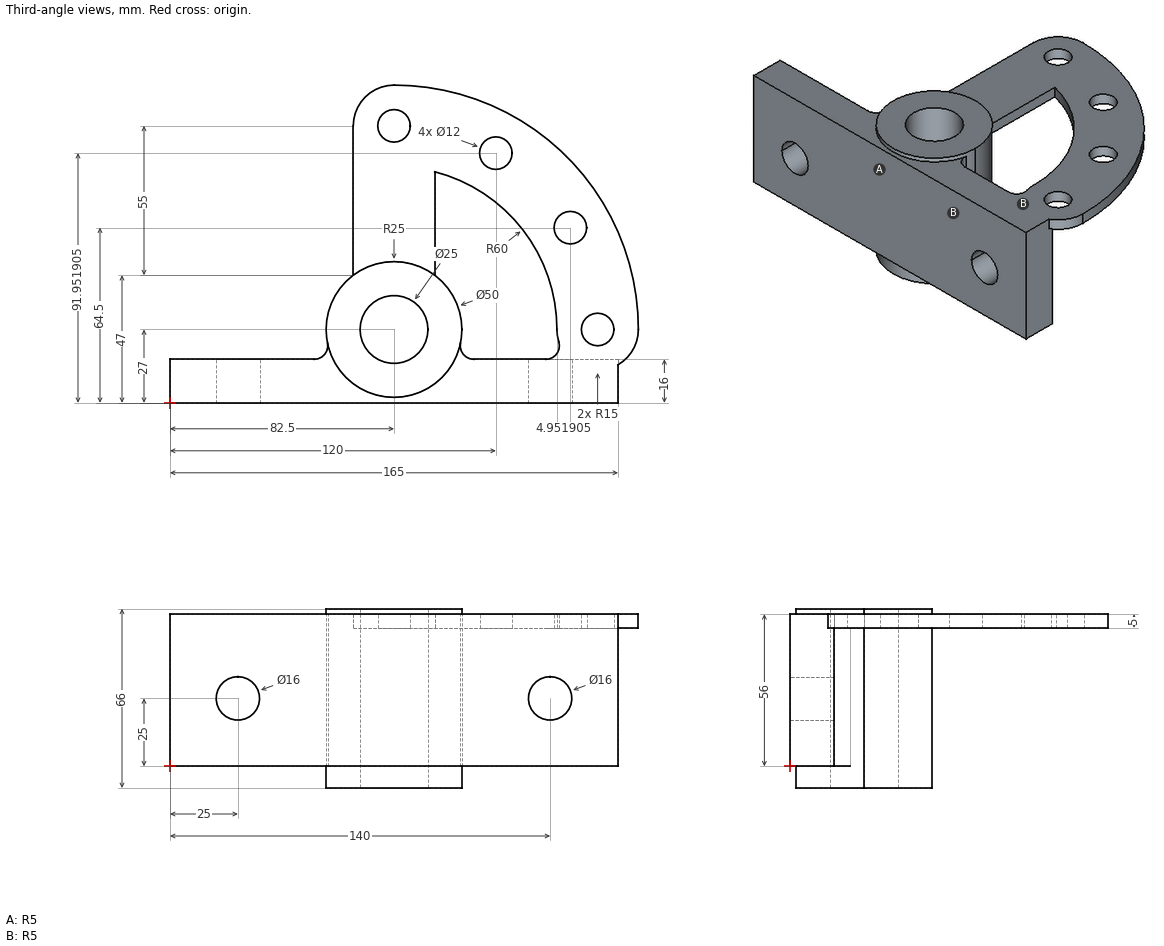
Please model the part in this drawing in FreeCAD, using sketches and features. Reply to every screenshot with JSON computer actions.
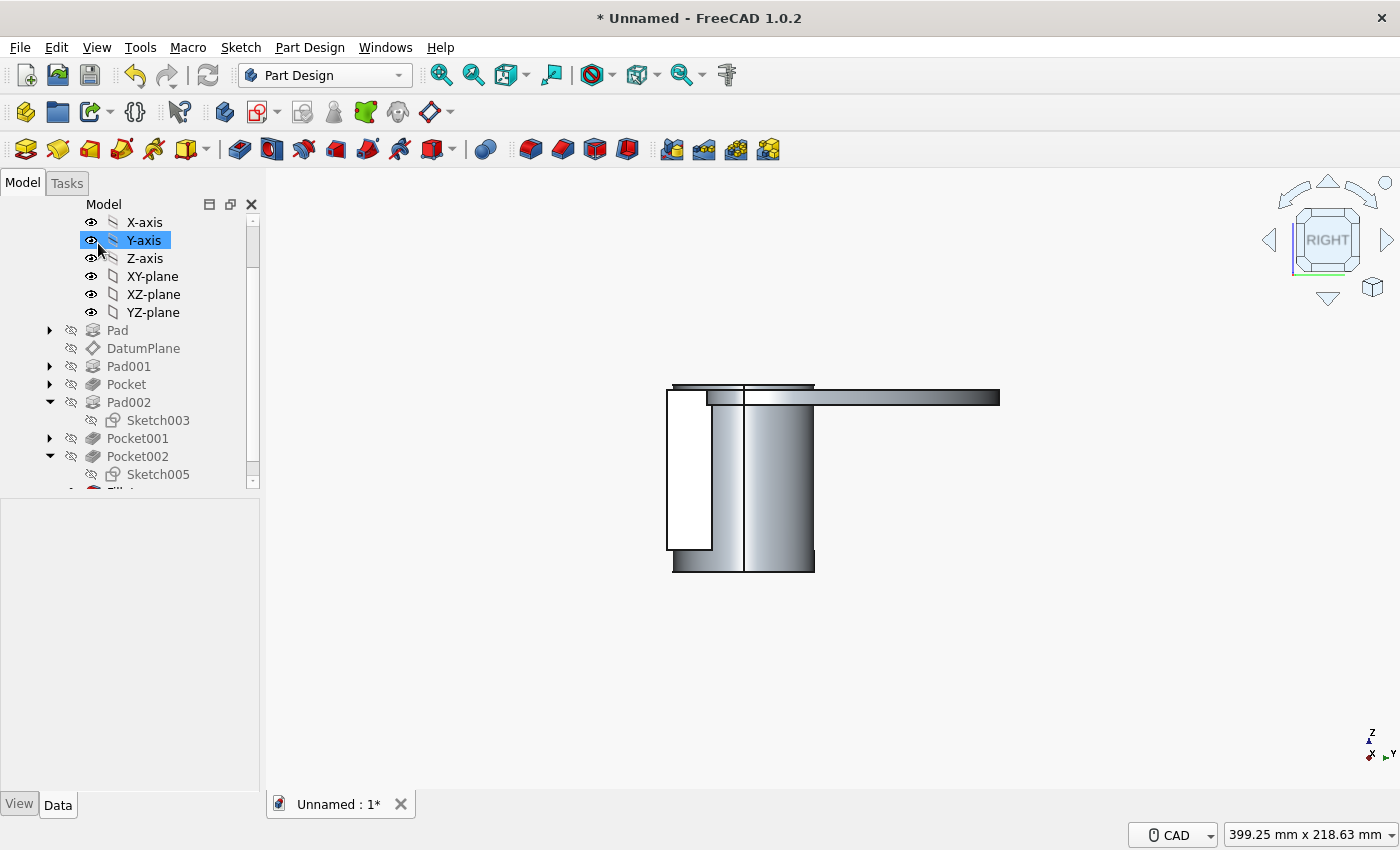
{"action": "key", "text": "5"}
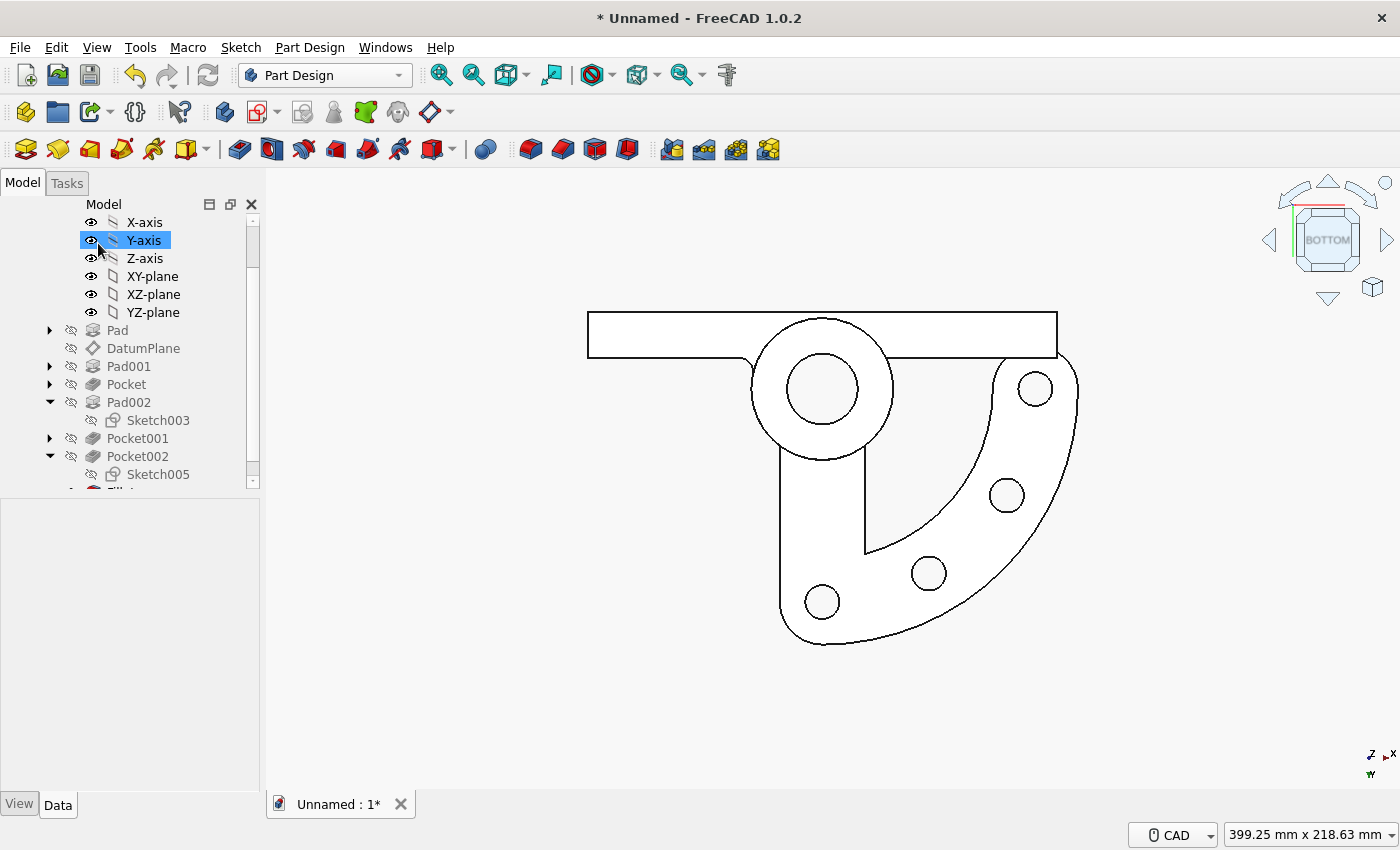
{"action": "key", "text": "4"}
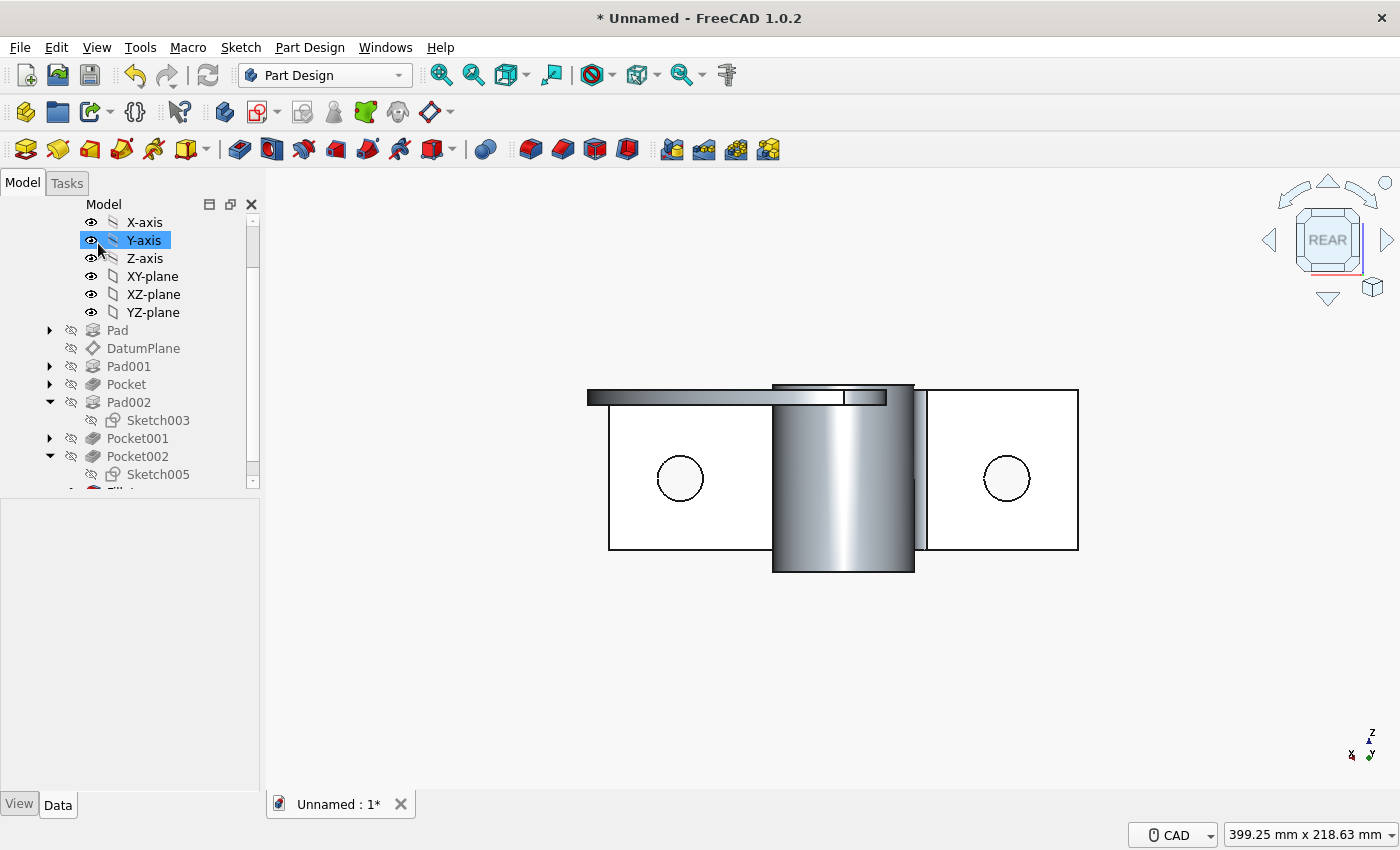
{"action": "left_click", "coordinate": [442, 76]}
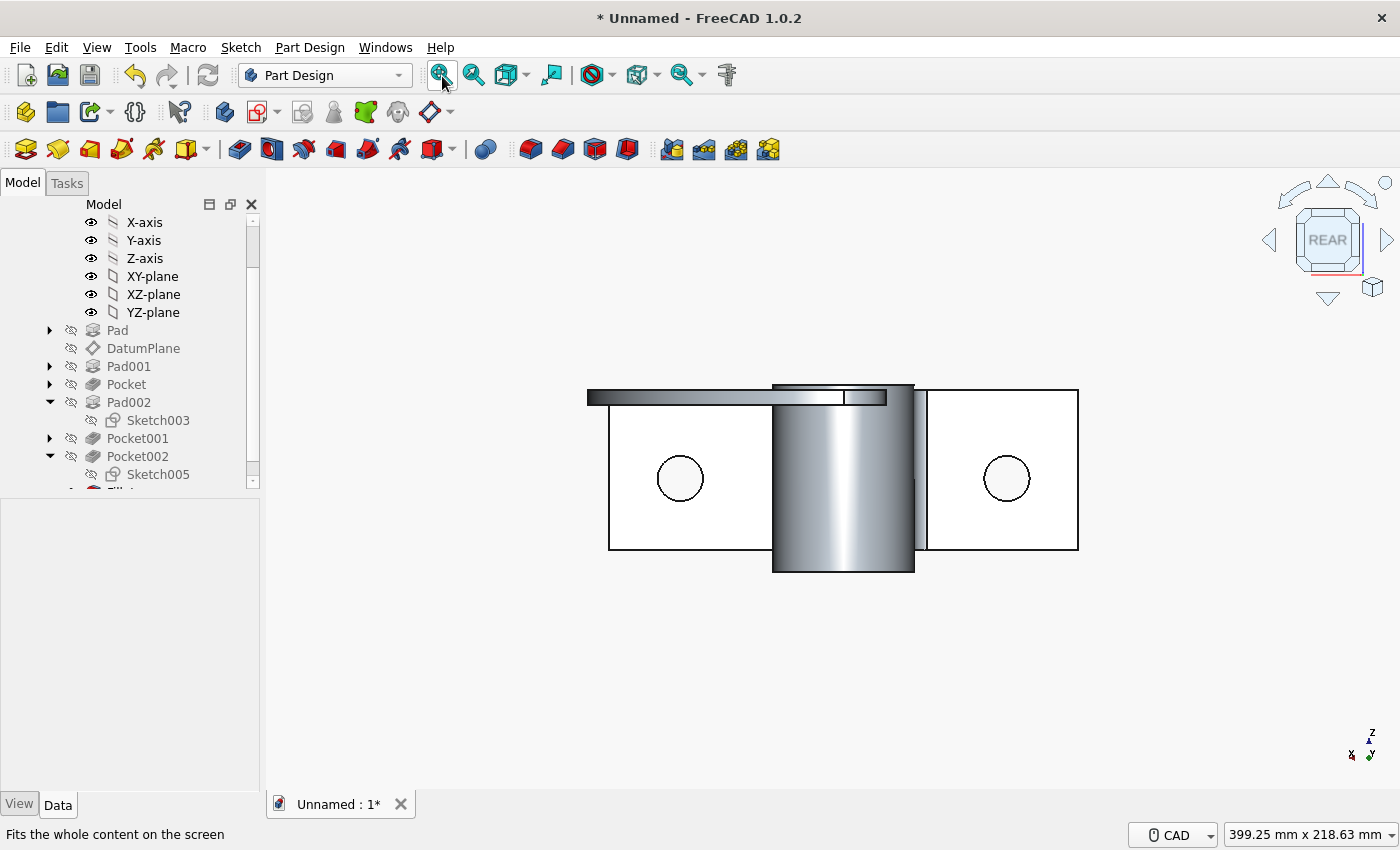
{"action": "key", "text": "6"}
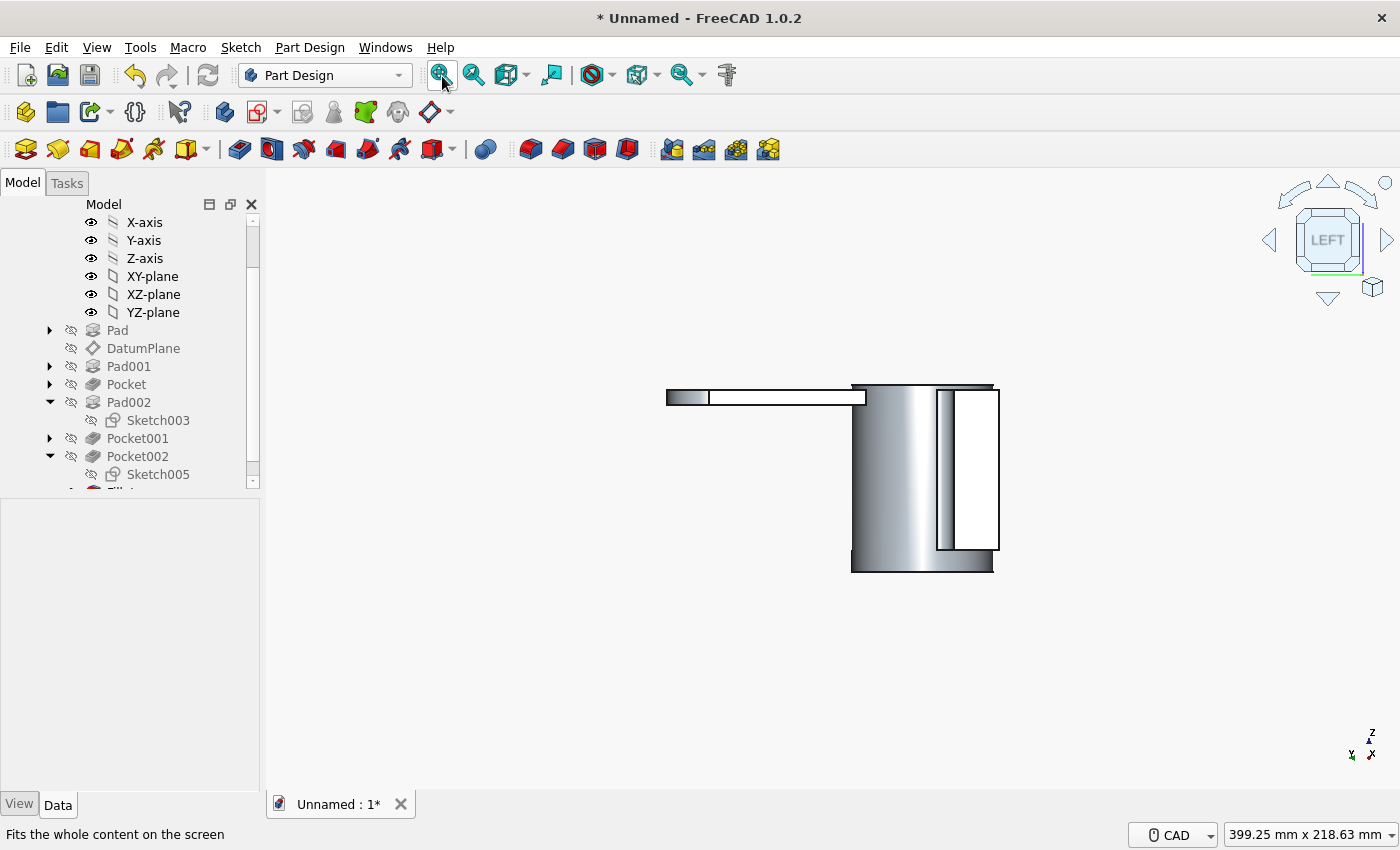
{"action": "left_click", "coordinate": [442, 76]}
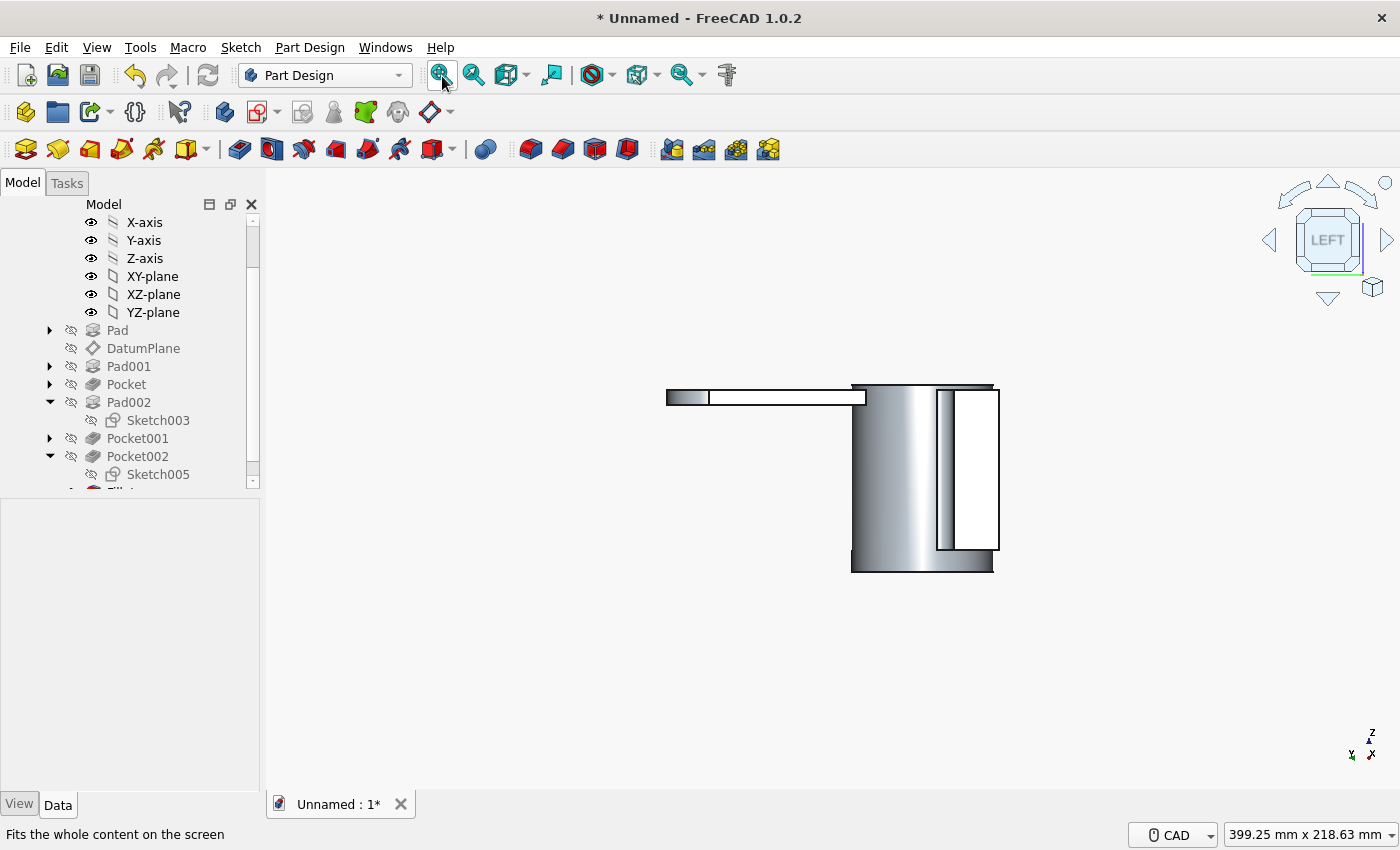
{"action": "key", "text": "v 3"}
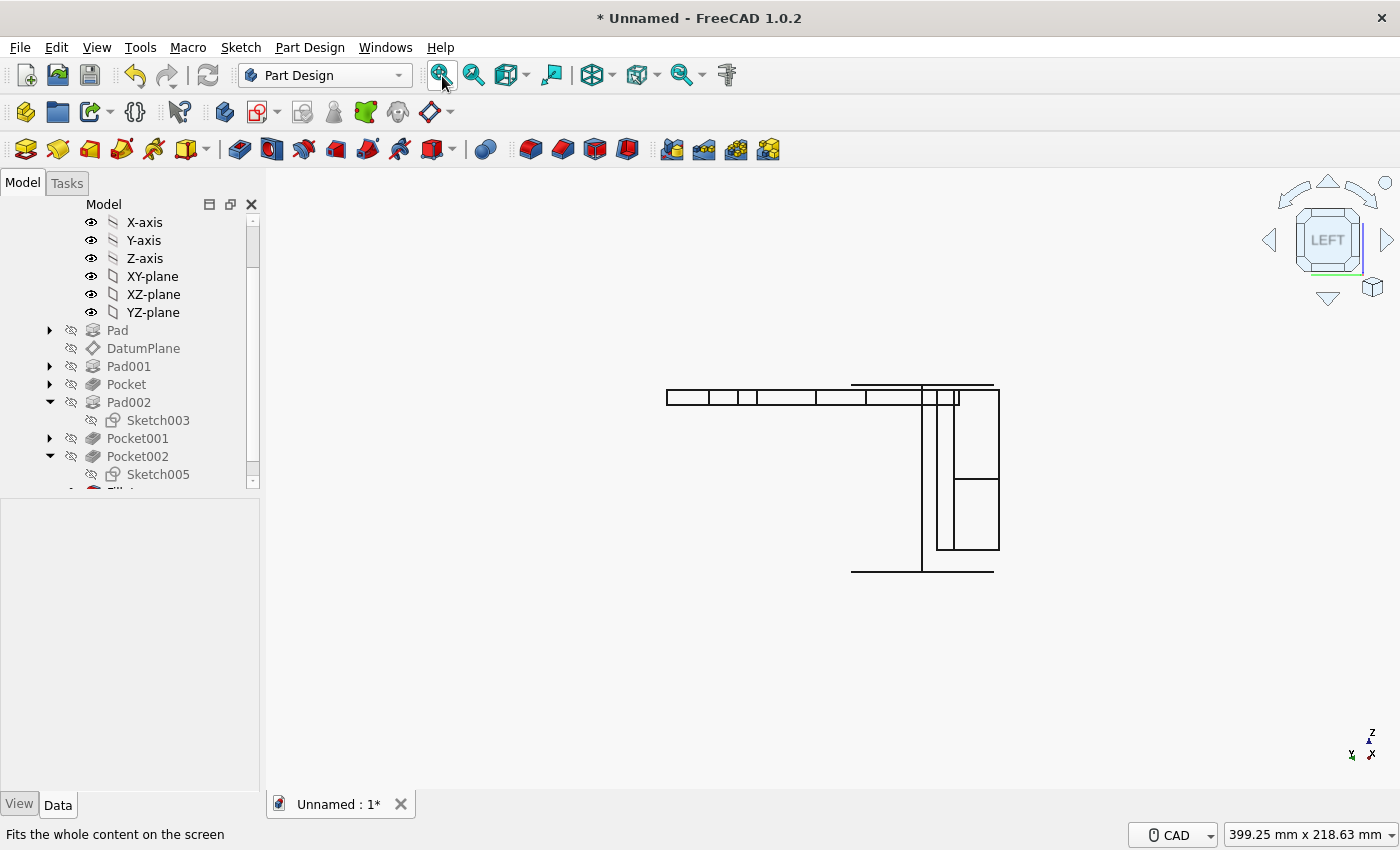
{"action": "key", "text": "0"}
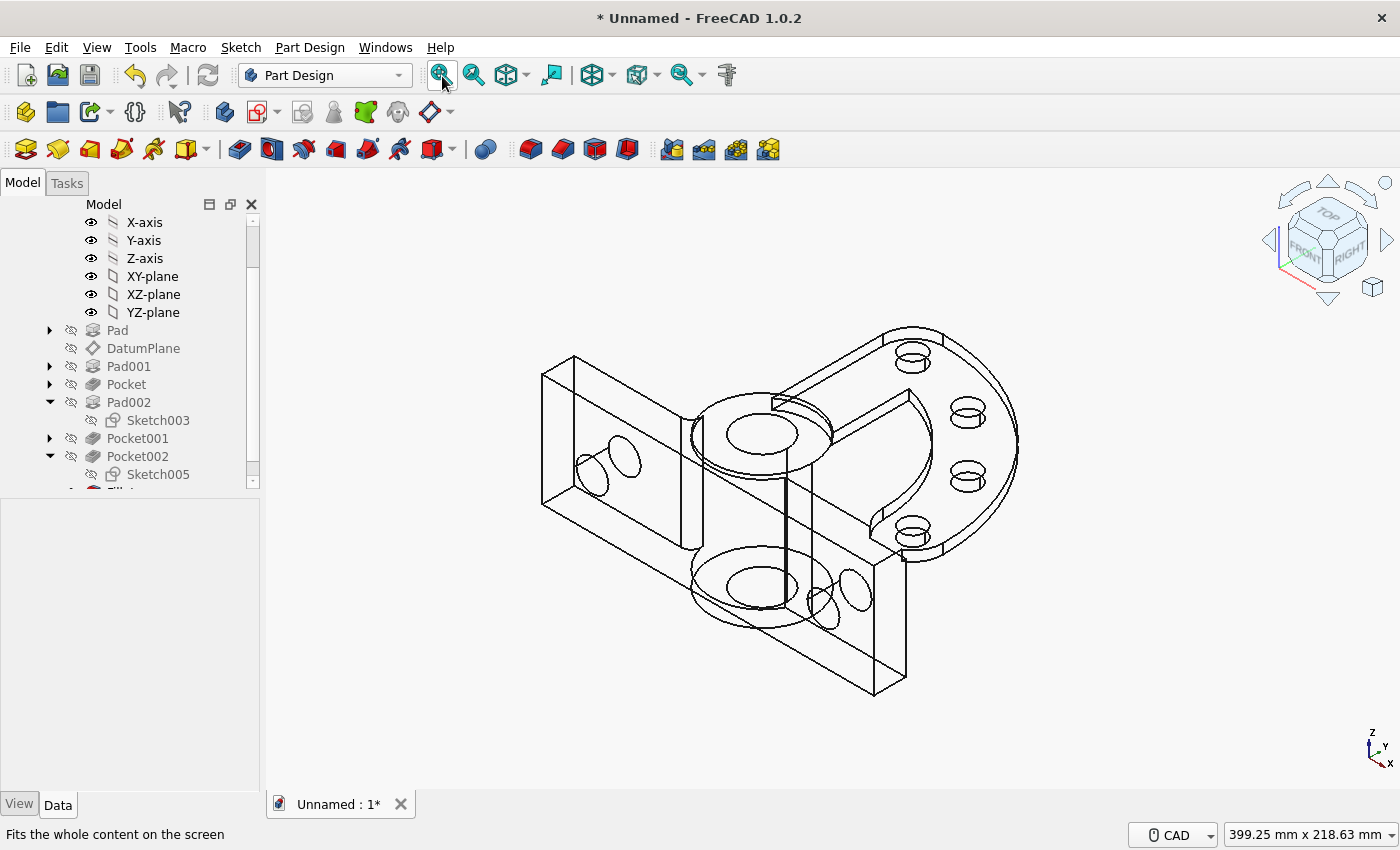
{"action": "left_click", "coordinate": [785, 542]}